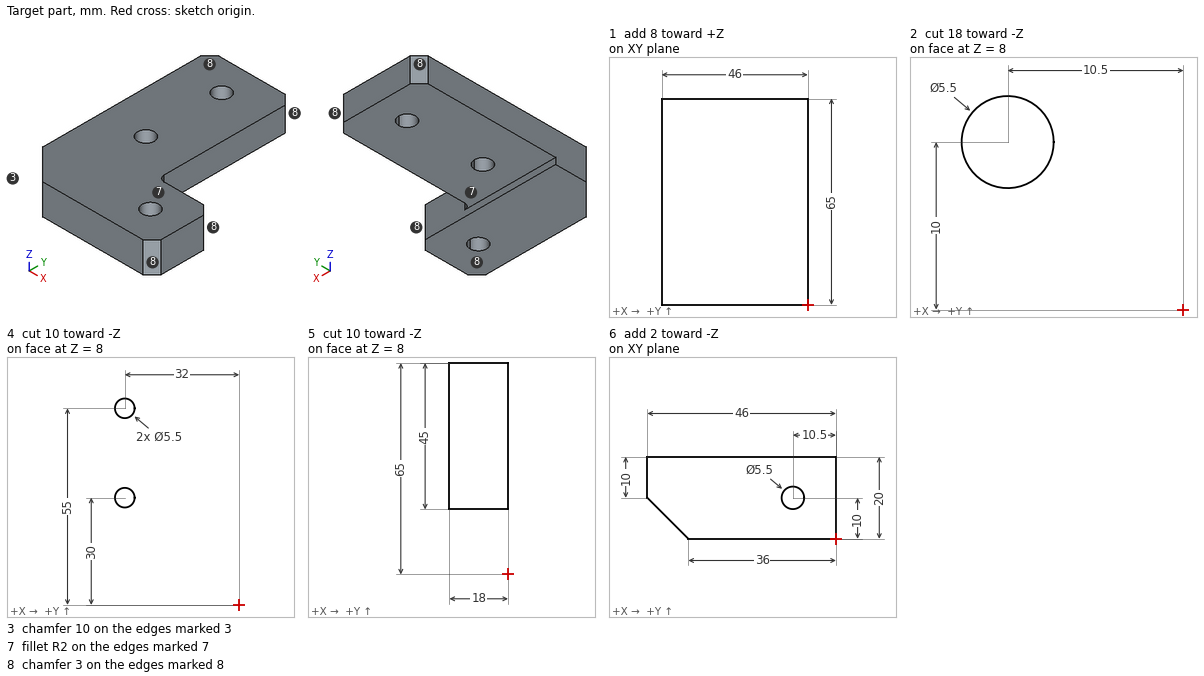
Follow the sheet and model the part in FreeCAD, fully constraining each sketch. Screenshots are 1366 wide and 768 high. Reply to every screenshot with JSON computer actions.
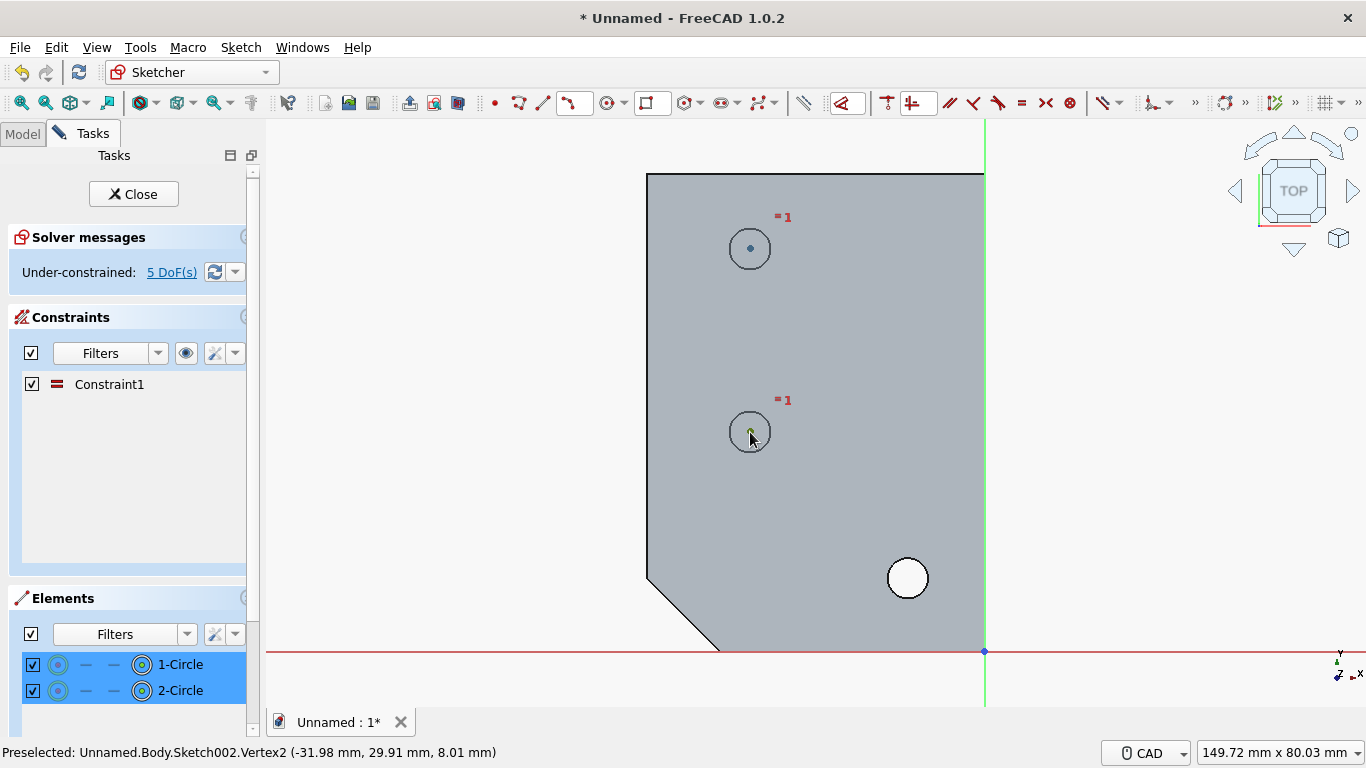
{"action": "left_click", "coordinate": [932, 104]}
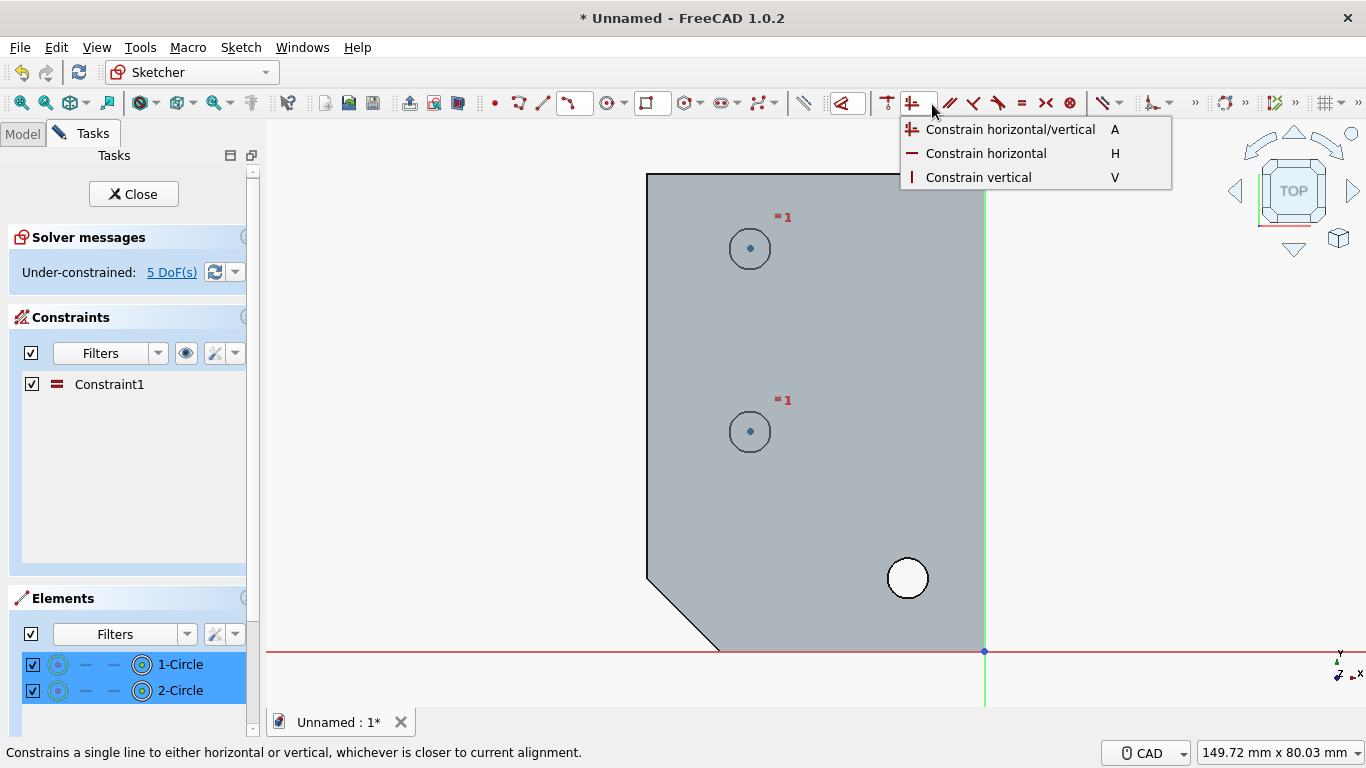
{"action": "left_click", "coordinate": [1036, 177]}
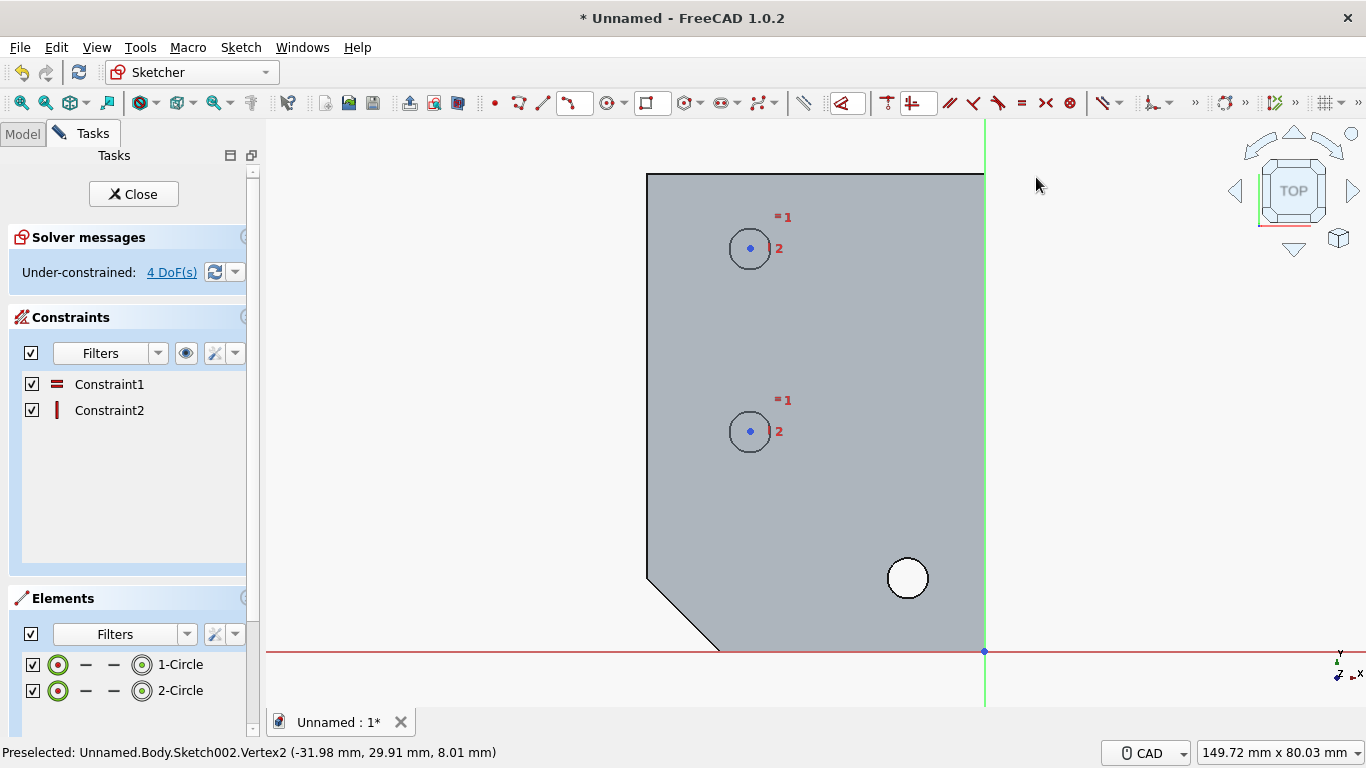
{"action": "left_click", "coordinate": [764, 234]}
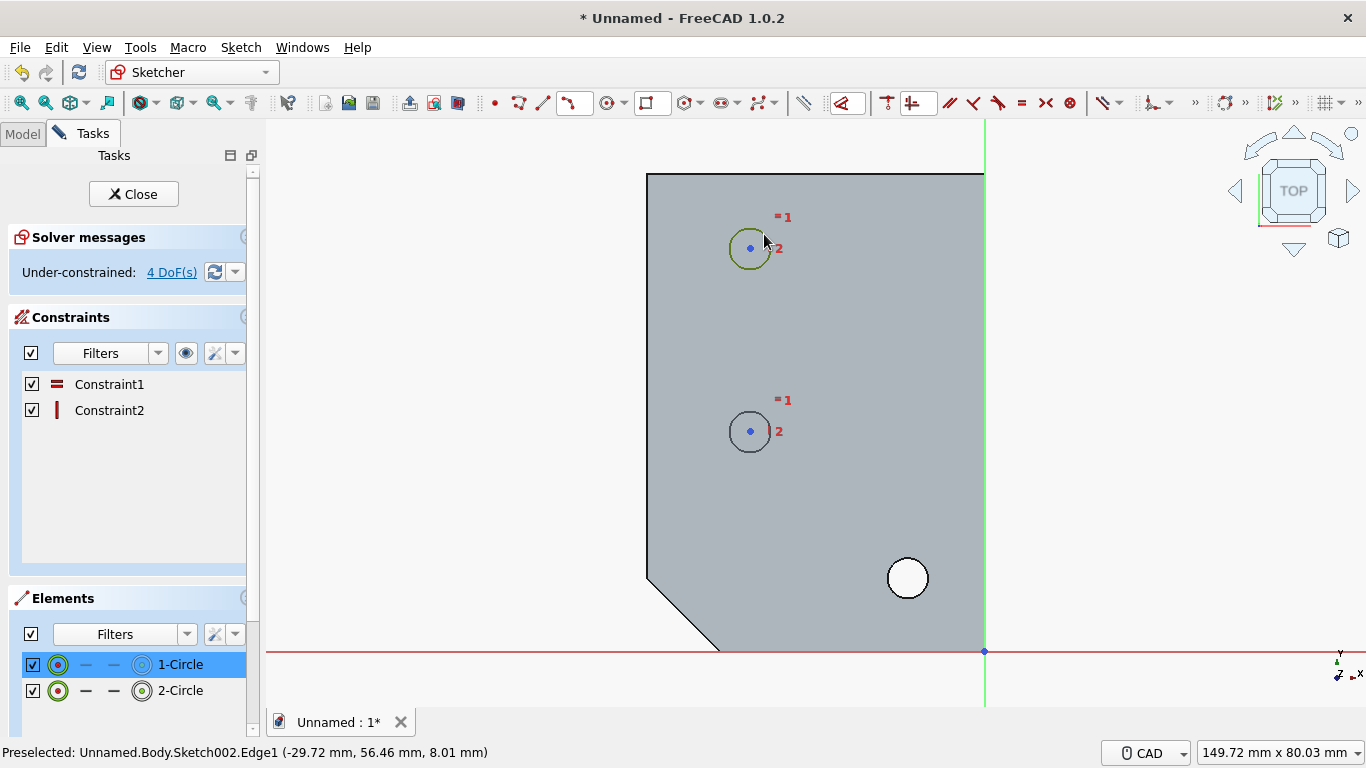
{"action": "key", "text": "k o"}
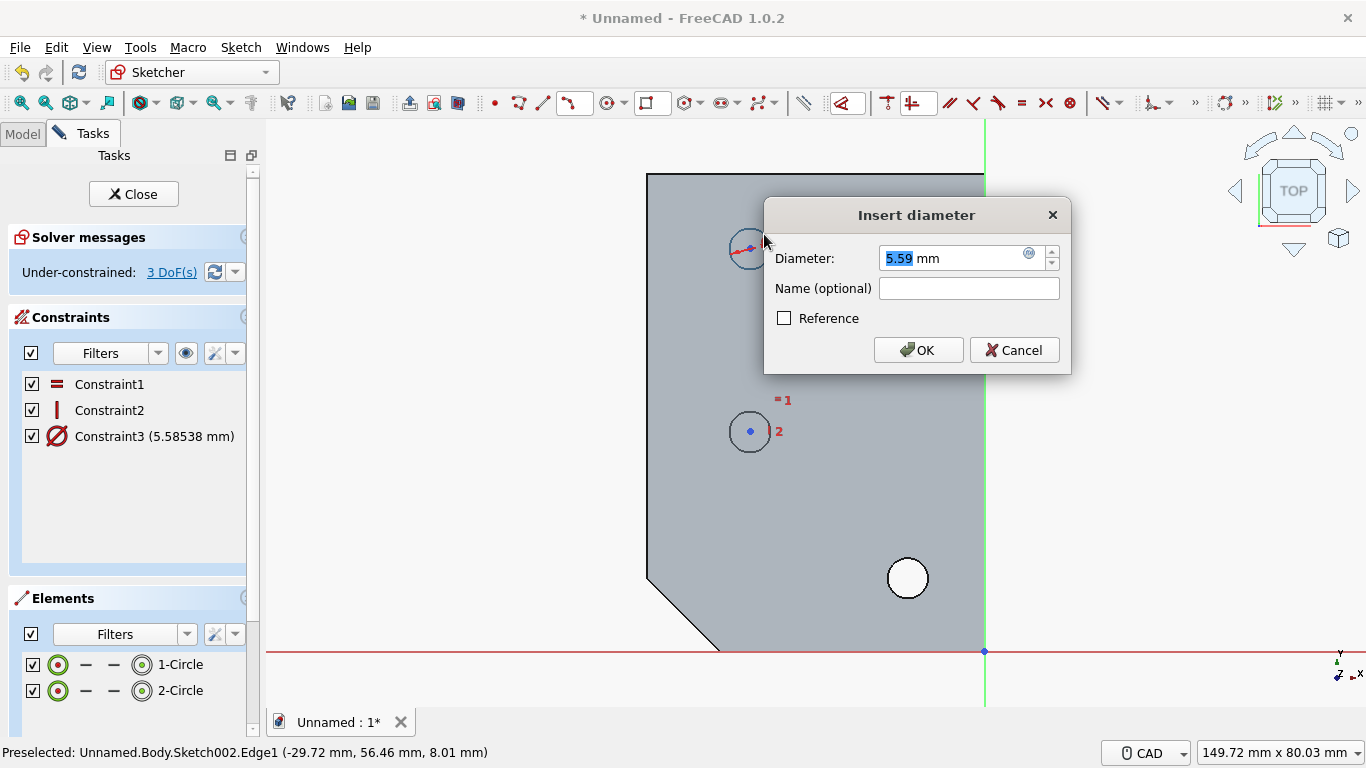
{"action": "type", "text": "5.5"}
{"action": "key", "text": "Return"}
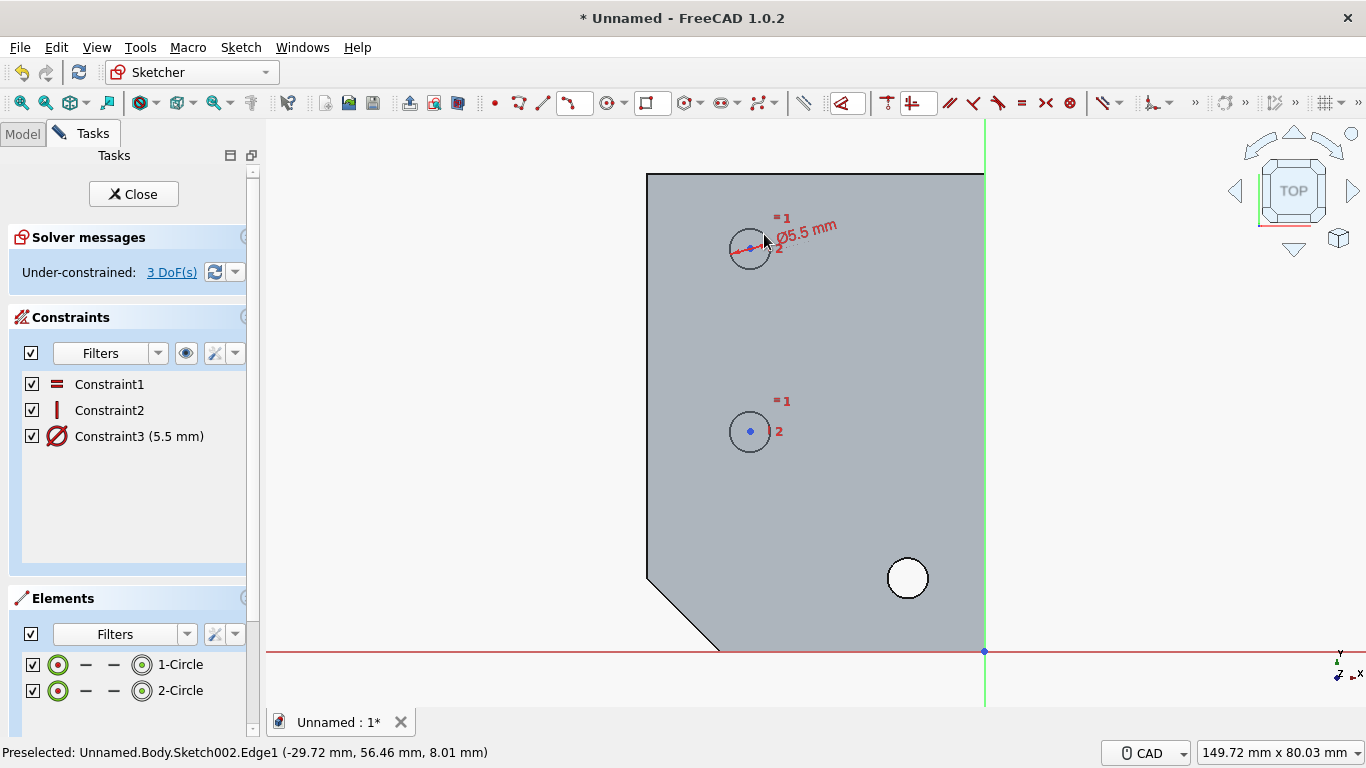
{"action": "left_click", "coordinate": [750, 249]}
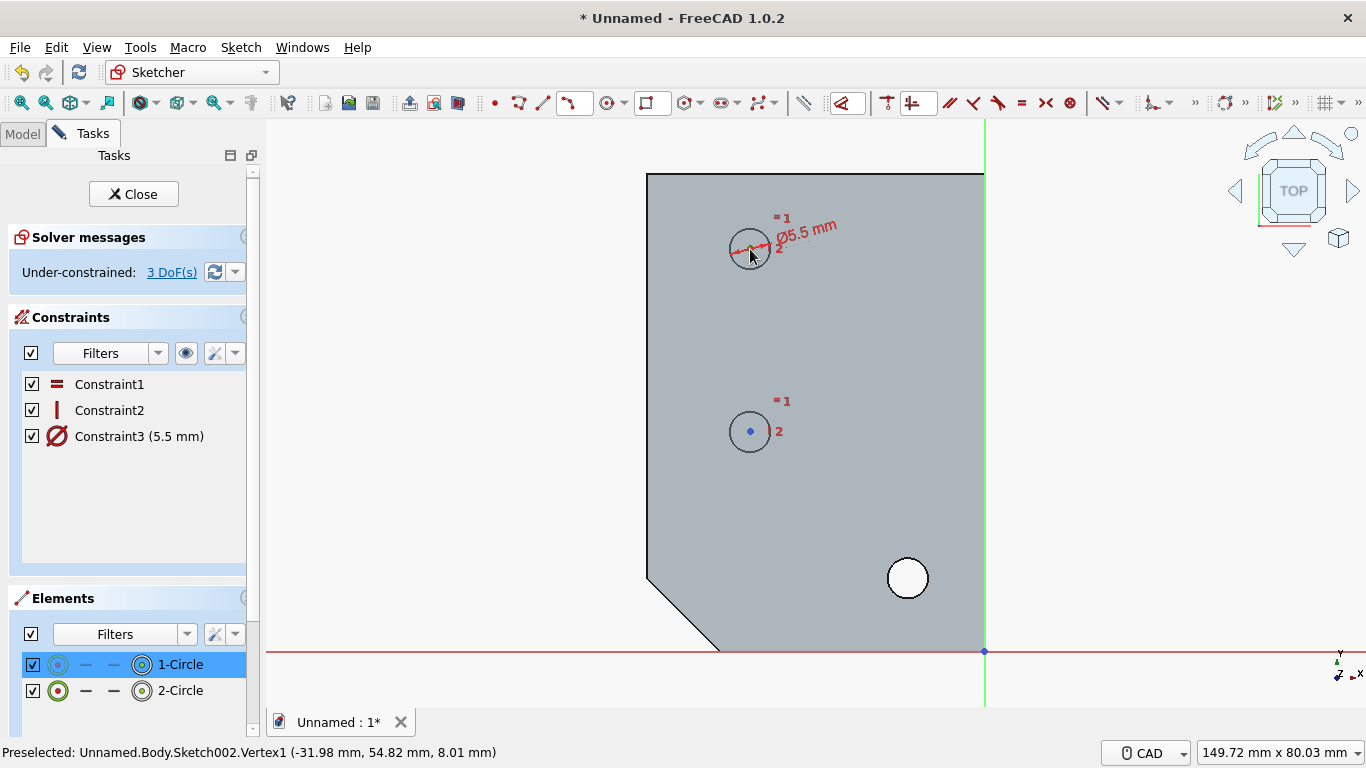
{"action": "left_click", "coordinate": [860, 104]}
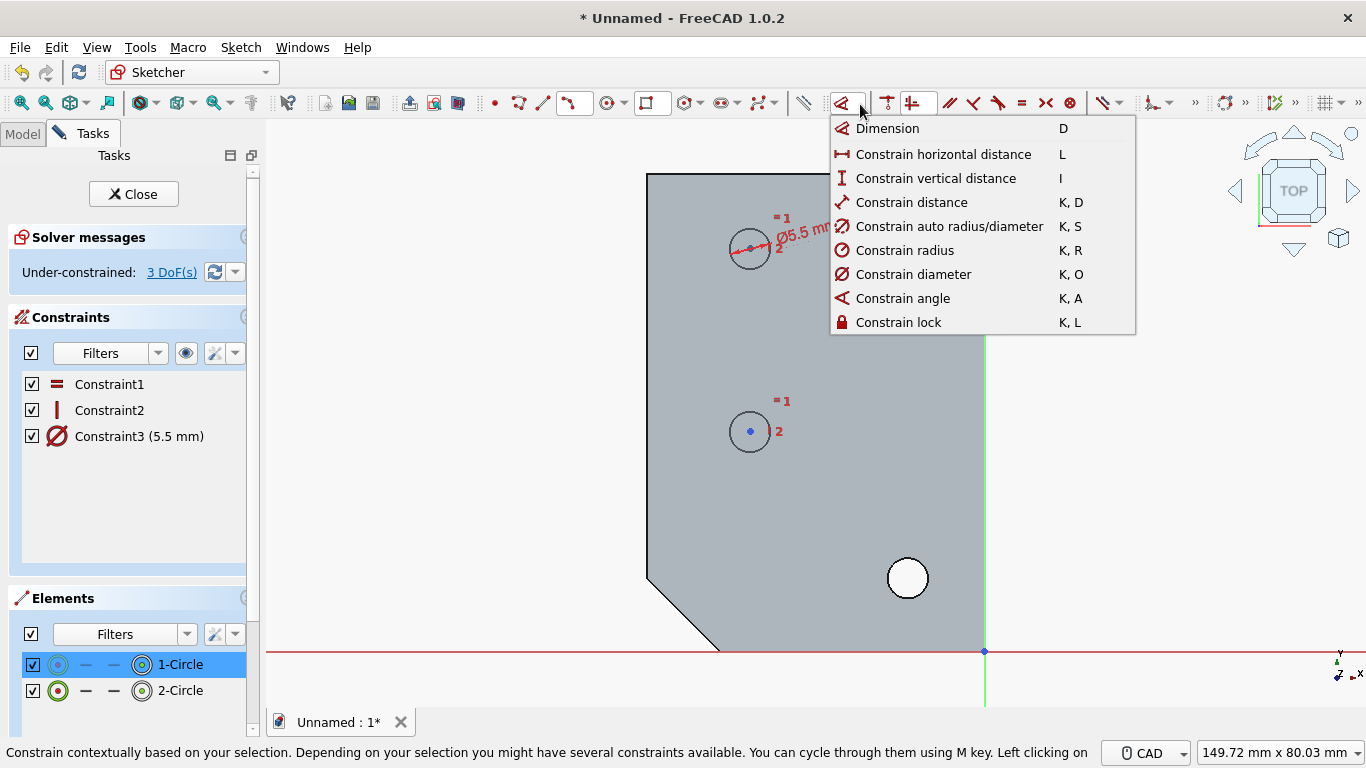
{"action": "left_click", "coordinate": [983, 154]}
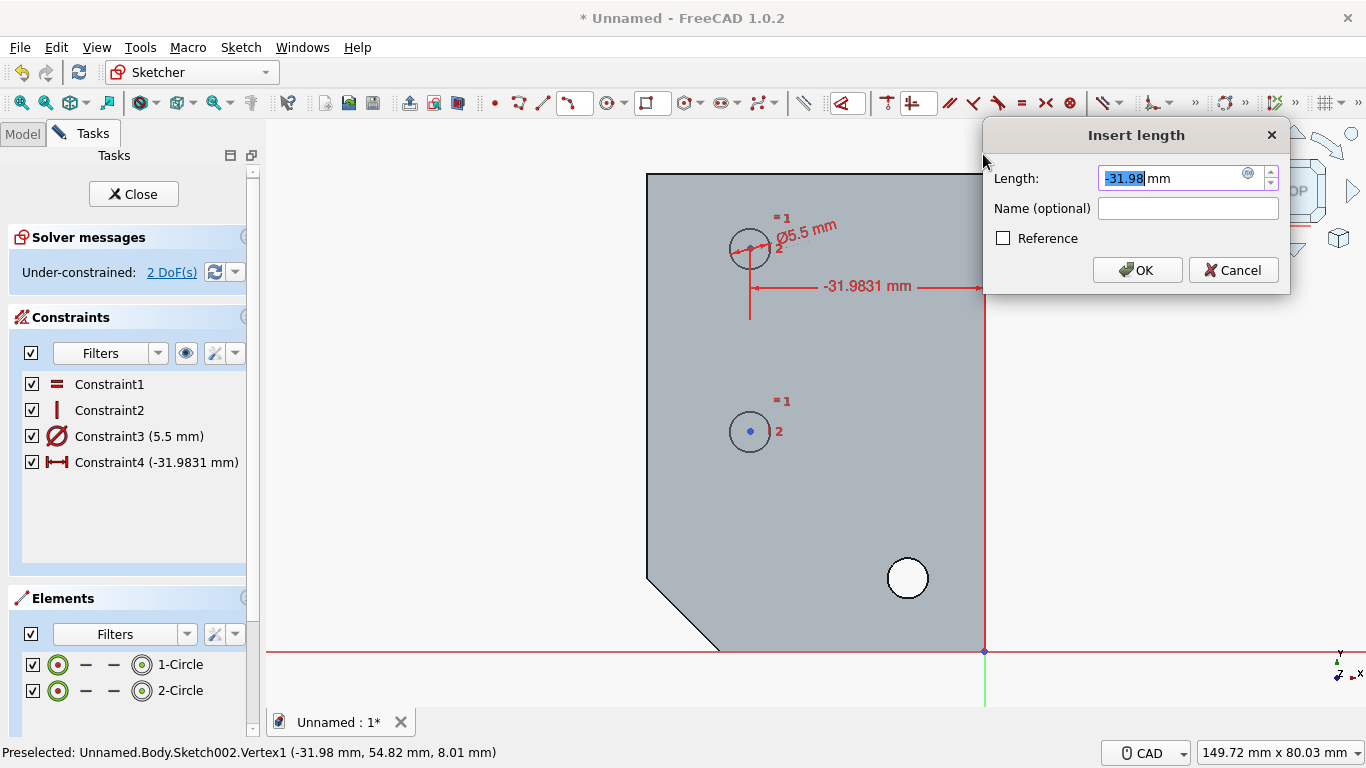
{"action": "type", "text": "-32"}
{"action": "key", "text": "Return"}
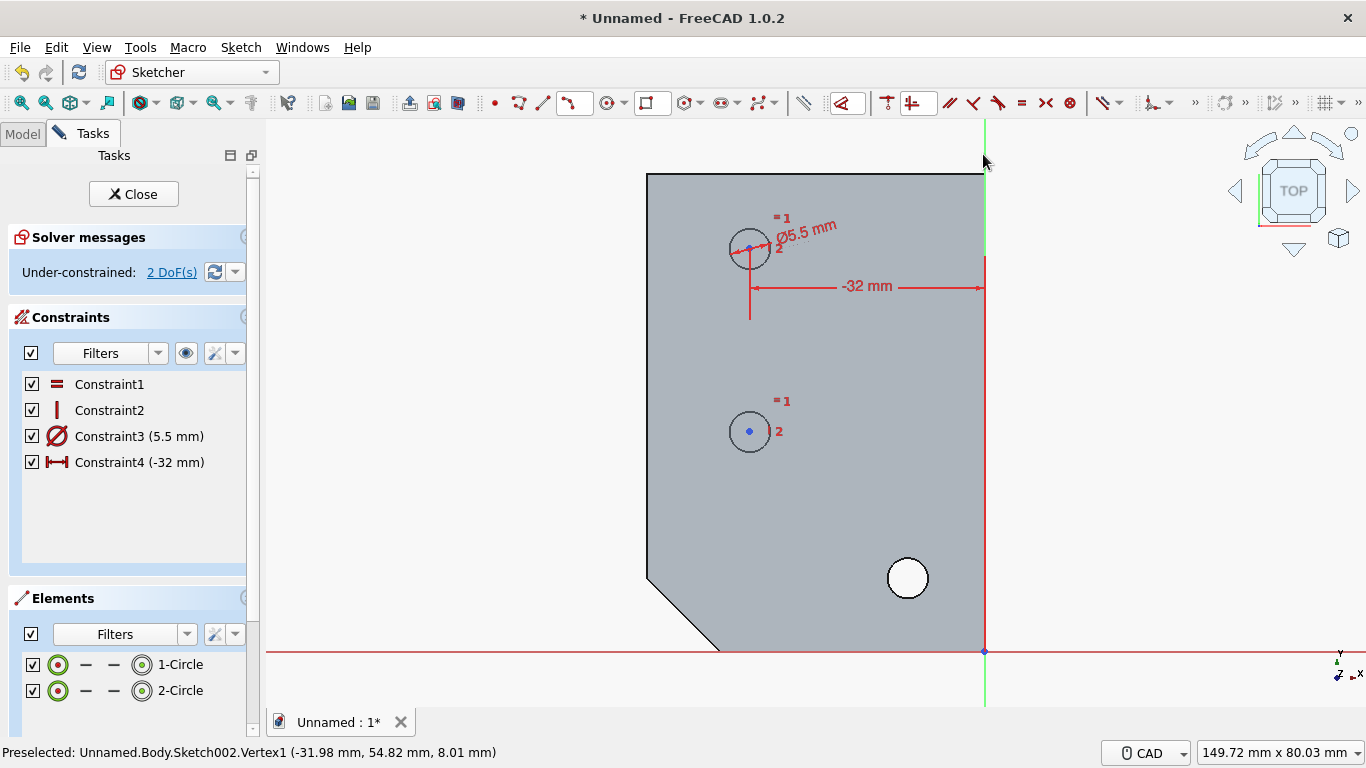
{"action": "left_click", "coordinate": [750, 249]}